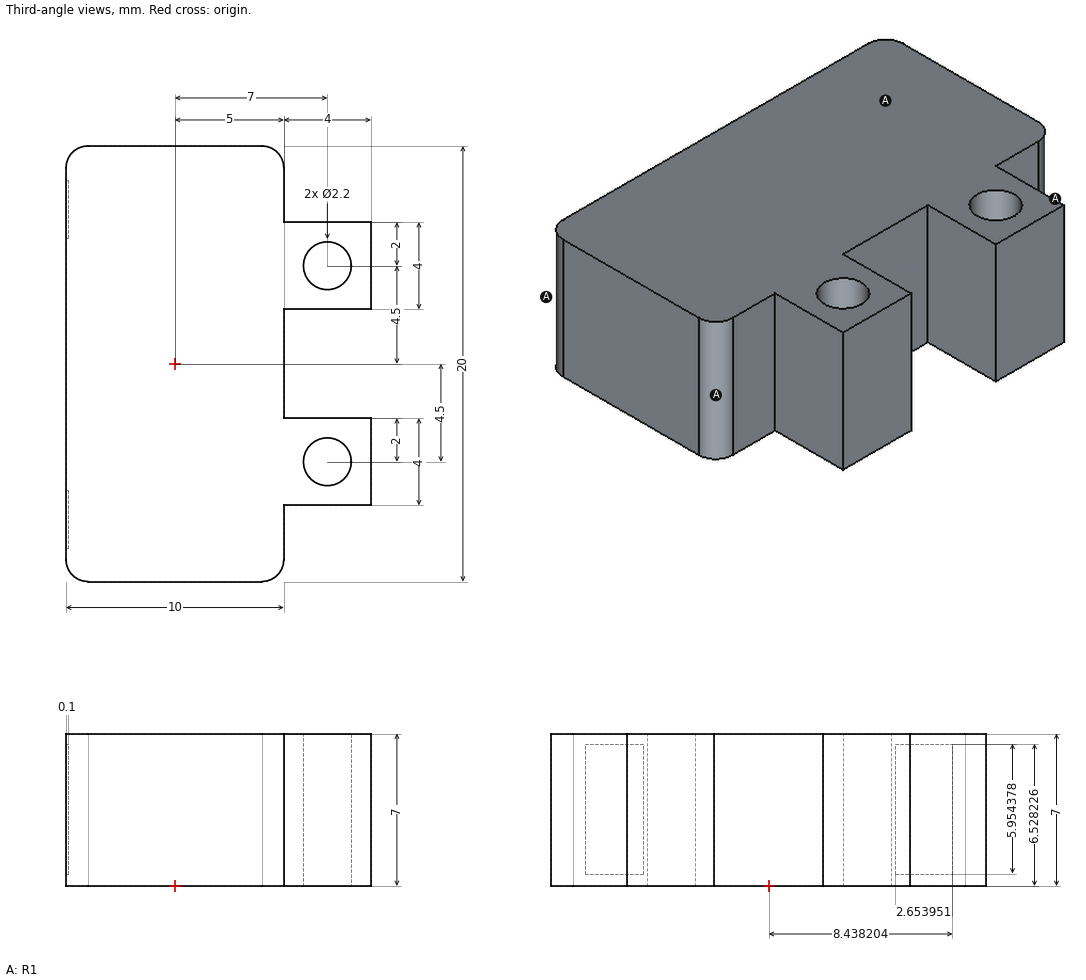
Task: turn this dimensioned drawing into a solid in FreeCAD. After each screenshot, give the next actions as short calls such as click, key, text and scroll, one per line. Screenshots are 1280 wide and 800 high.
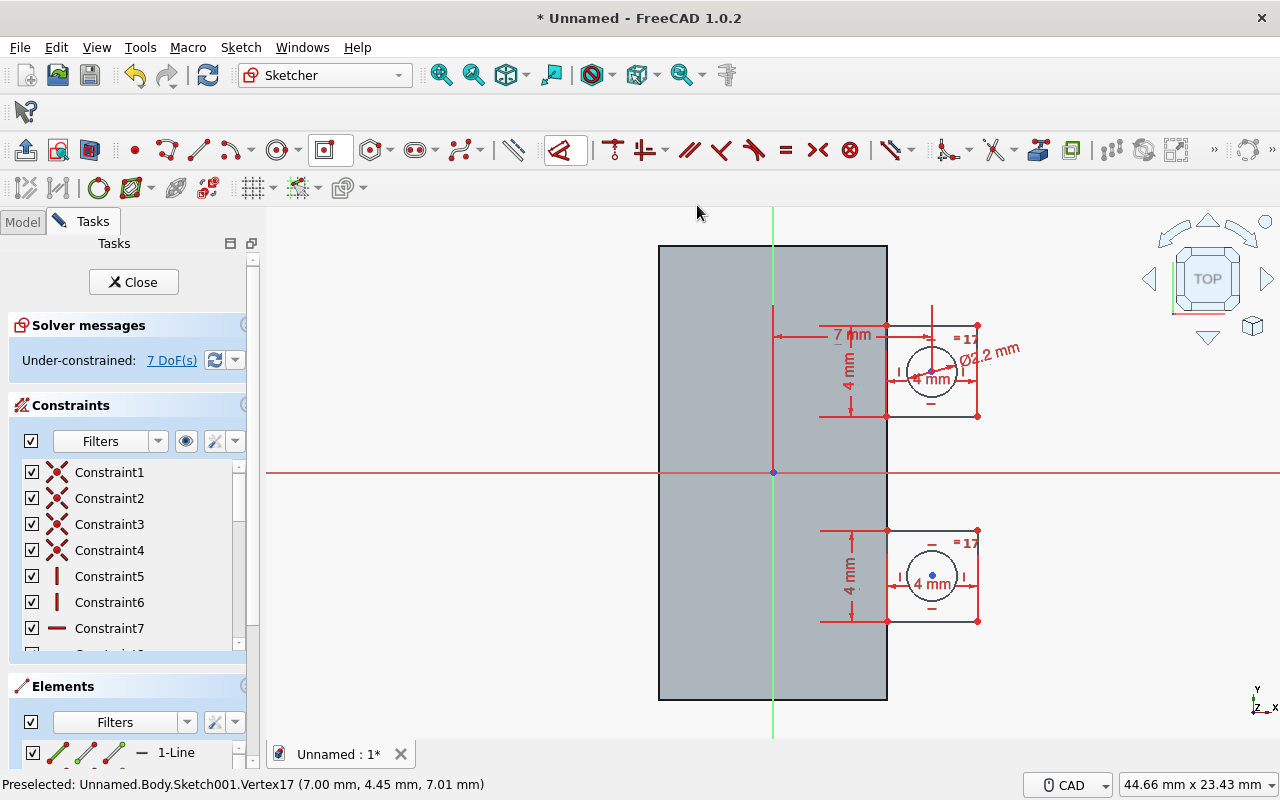
click(932, 576)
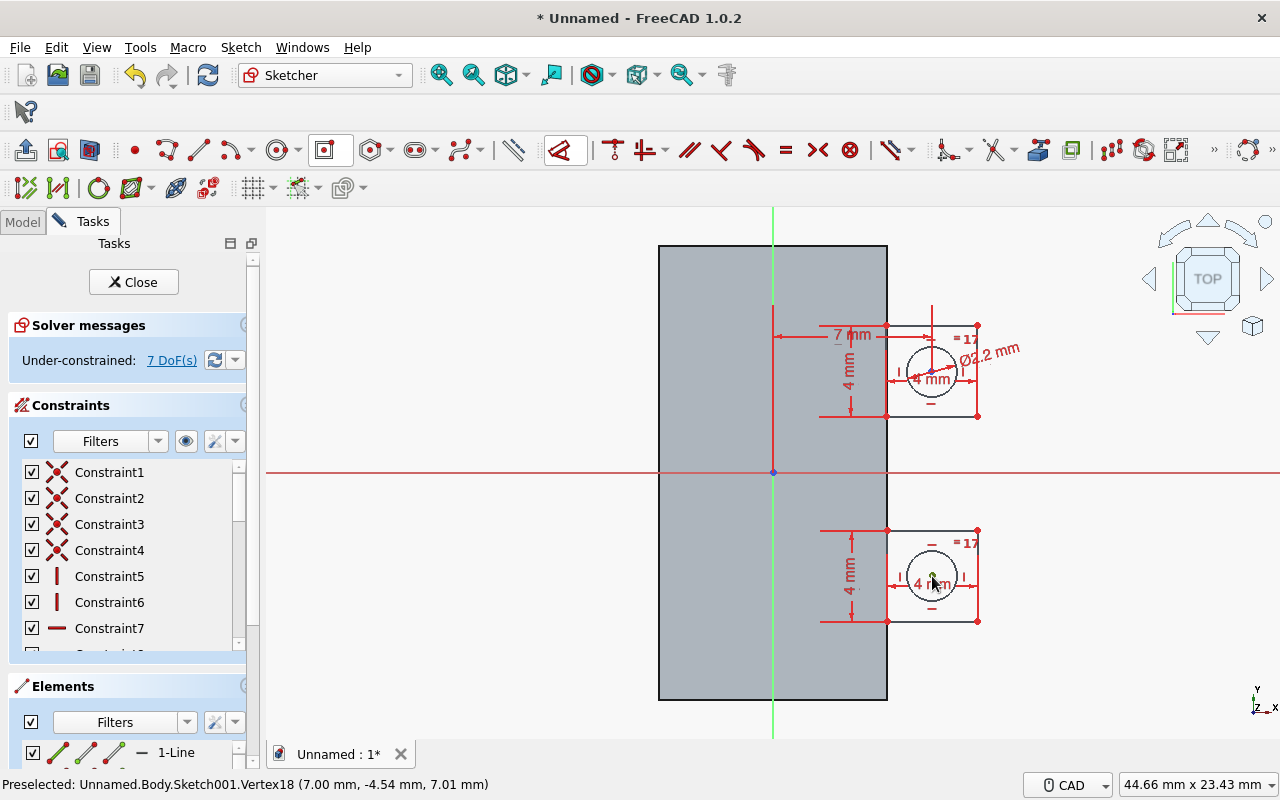
key(l)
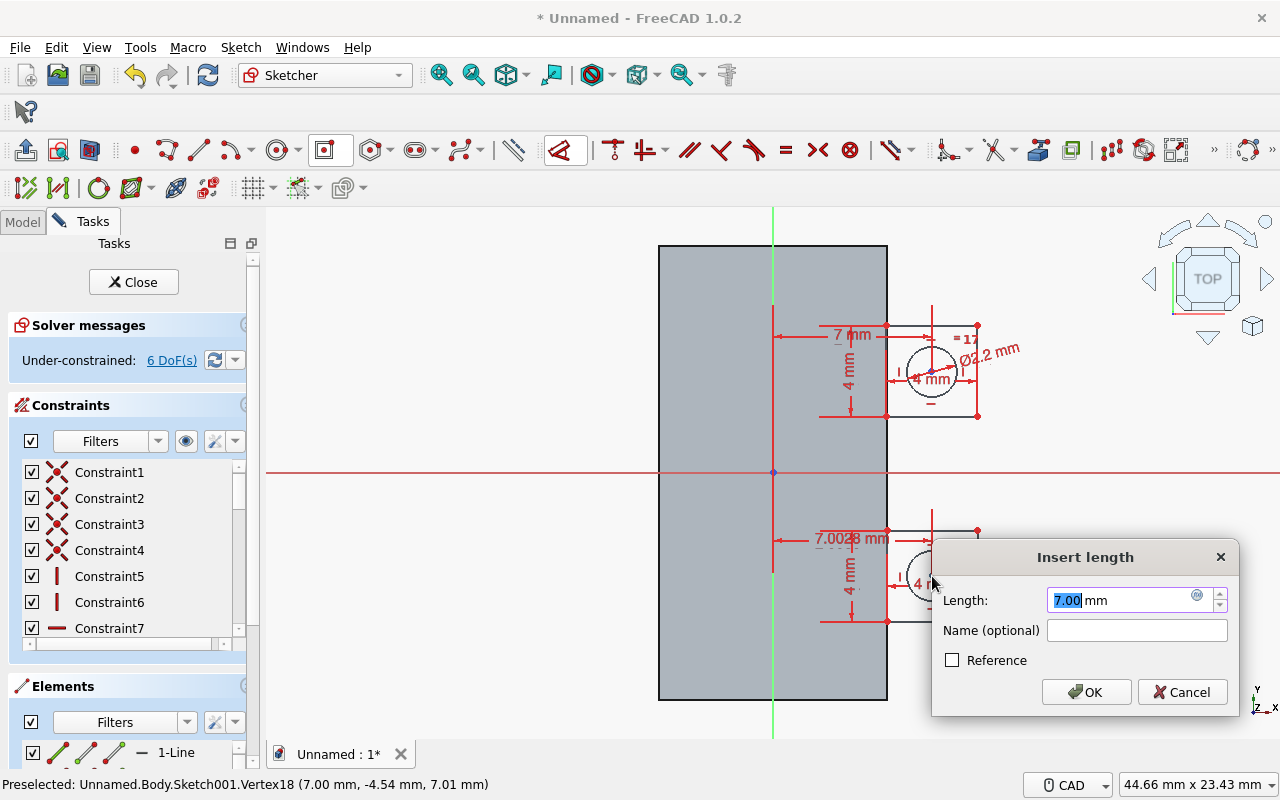
text(7)
key(Return)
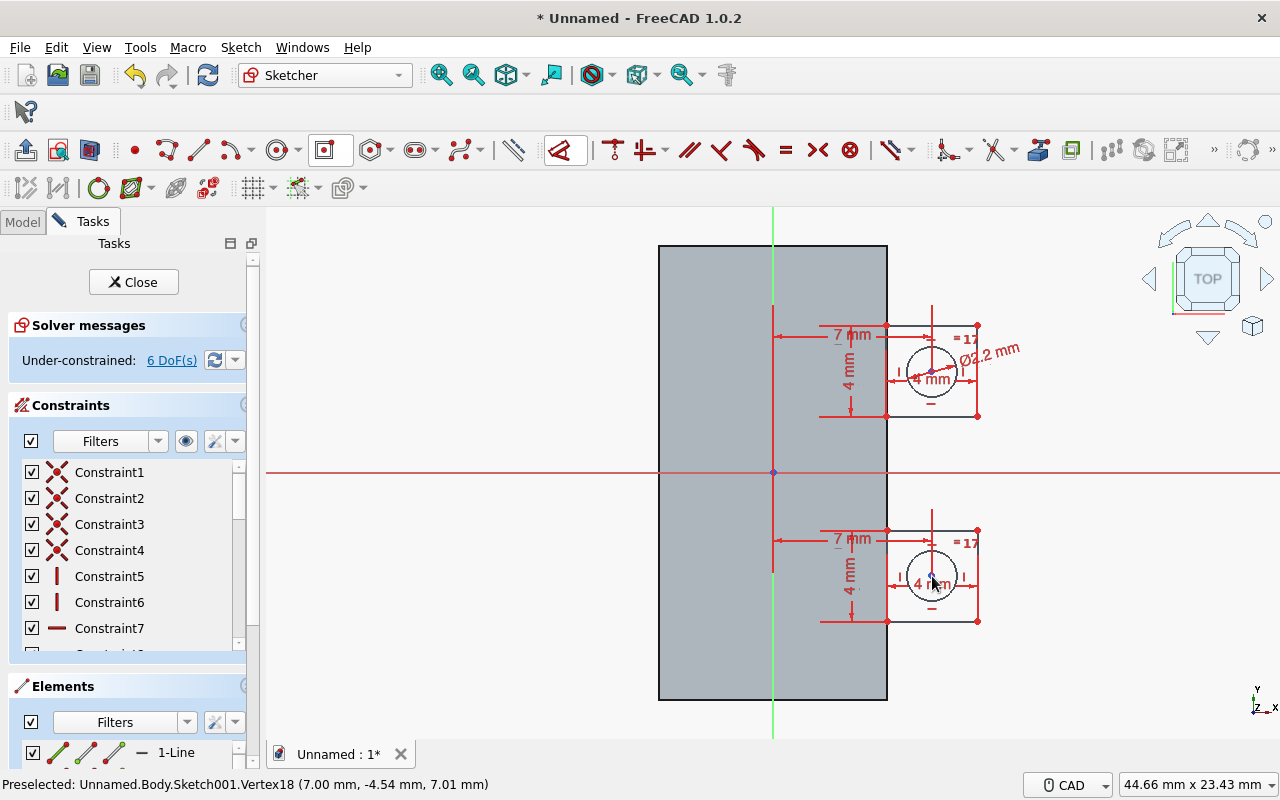
click(886, 326)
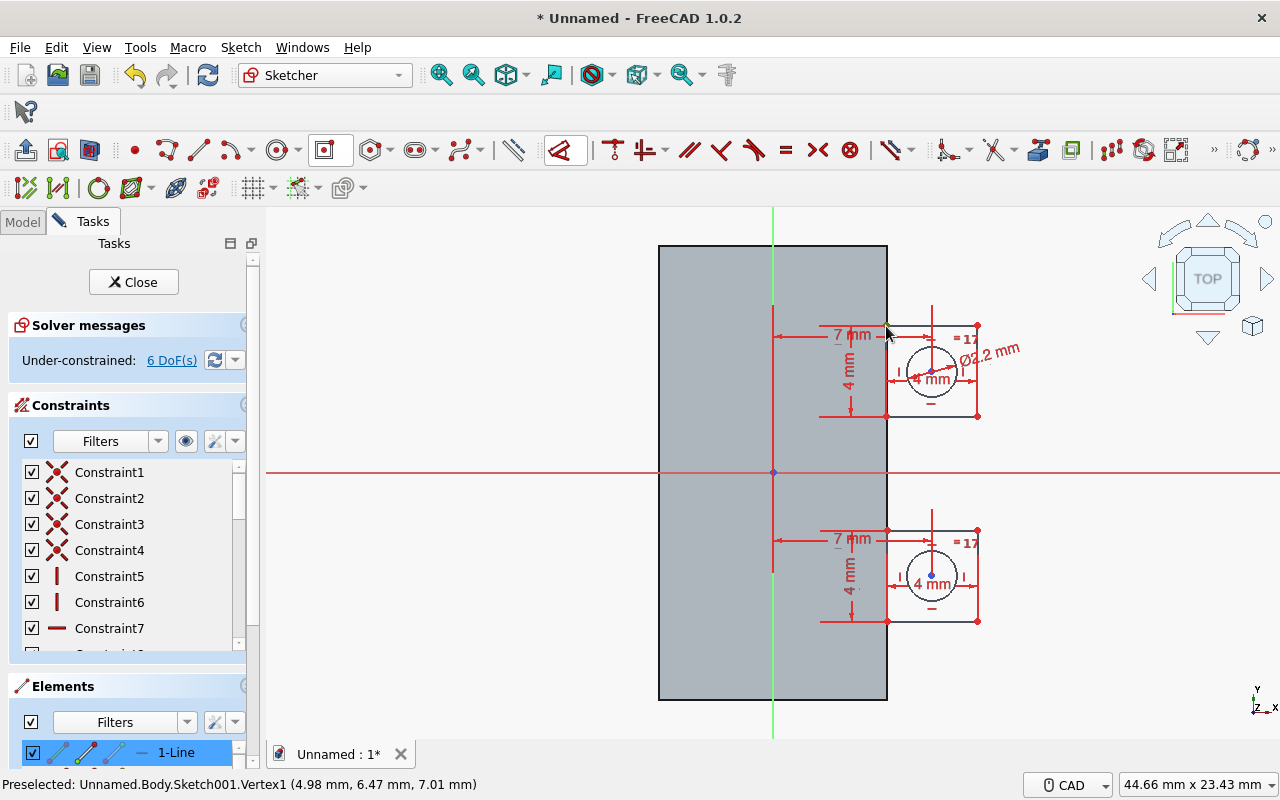
key(l)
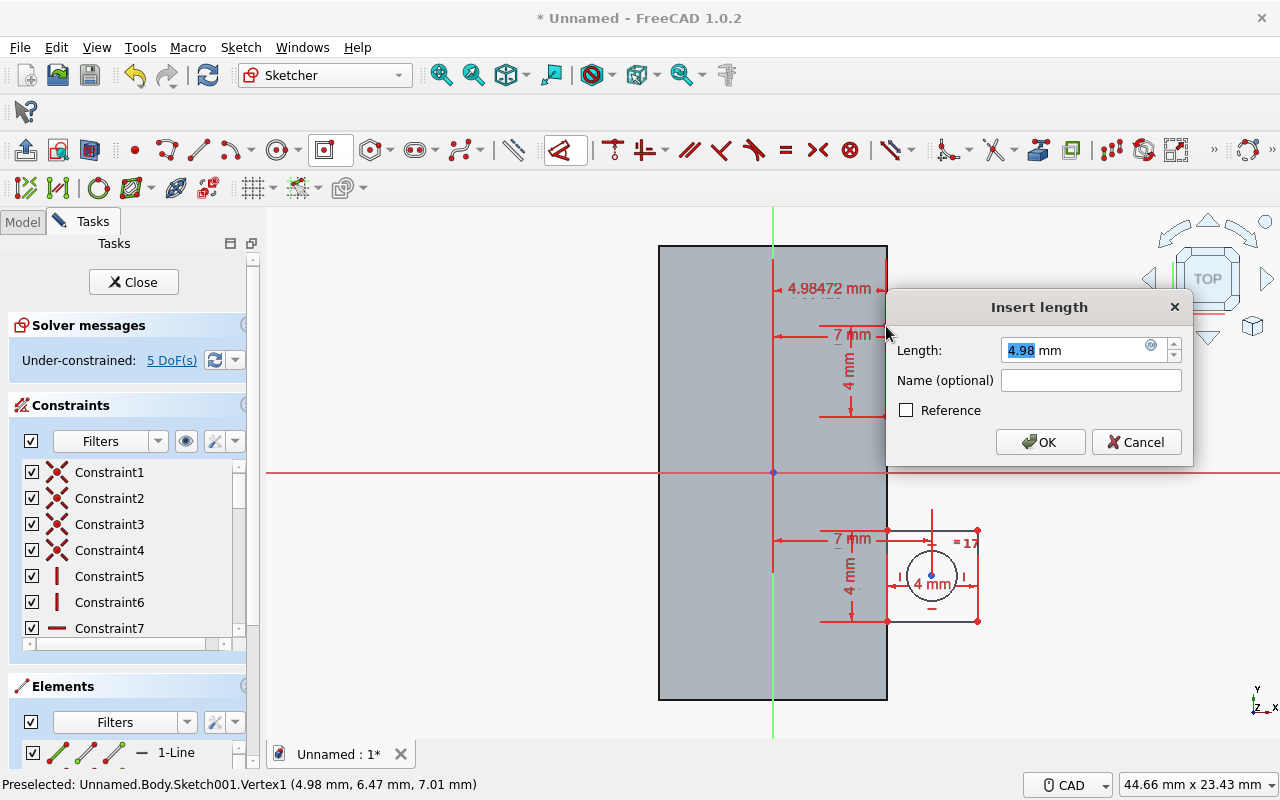
text(5)
key(Return)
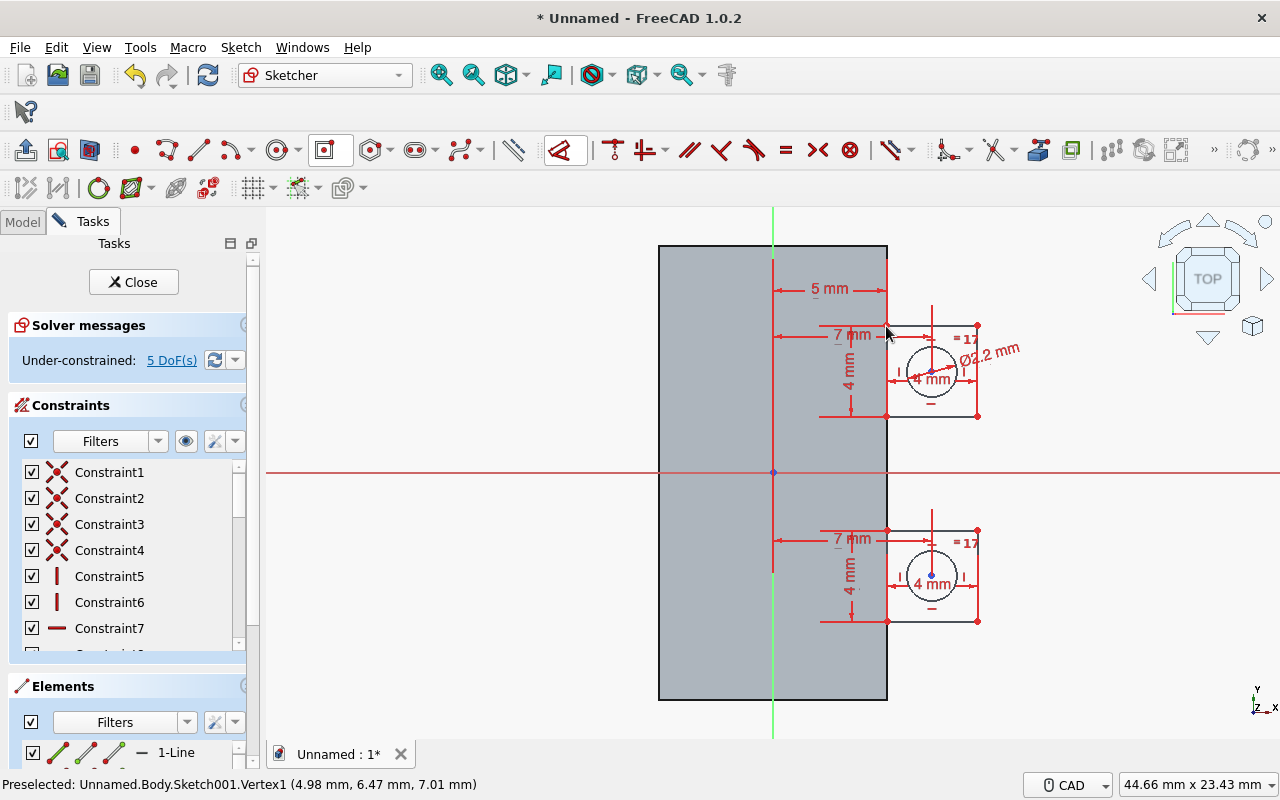
click(887, 531)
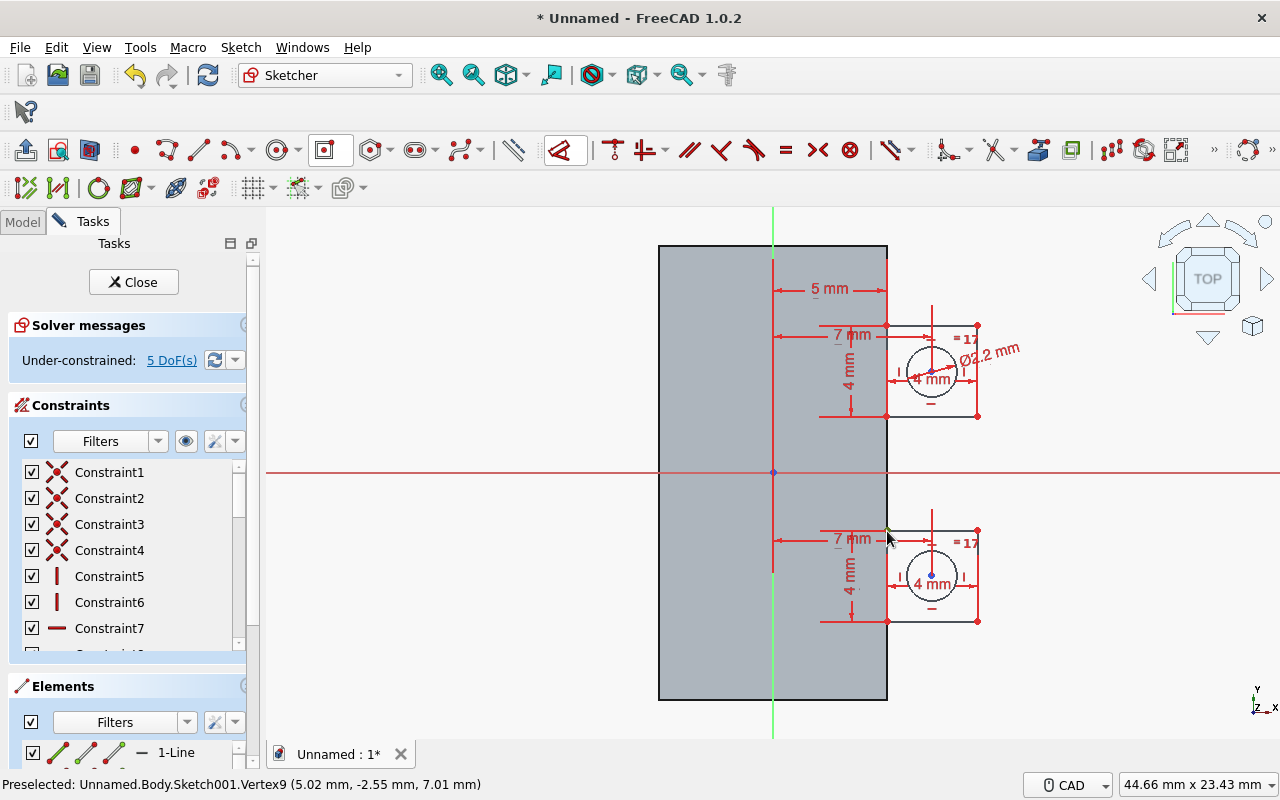
key(l)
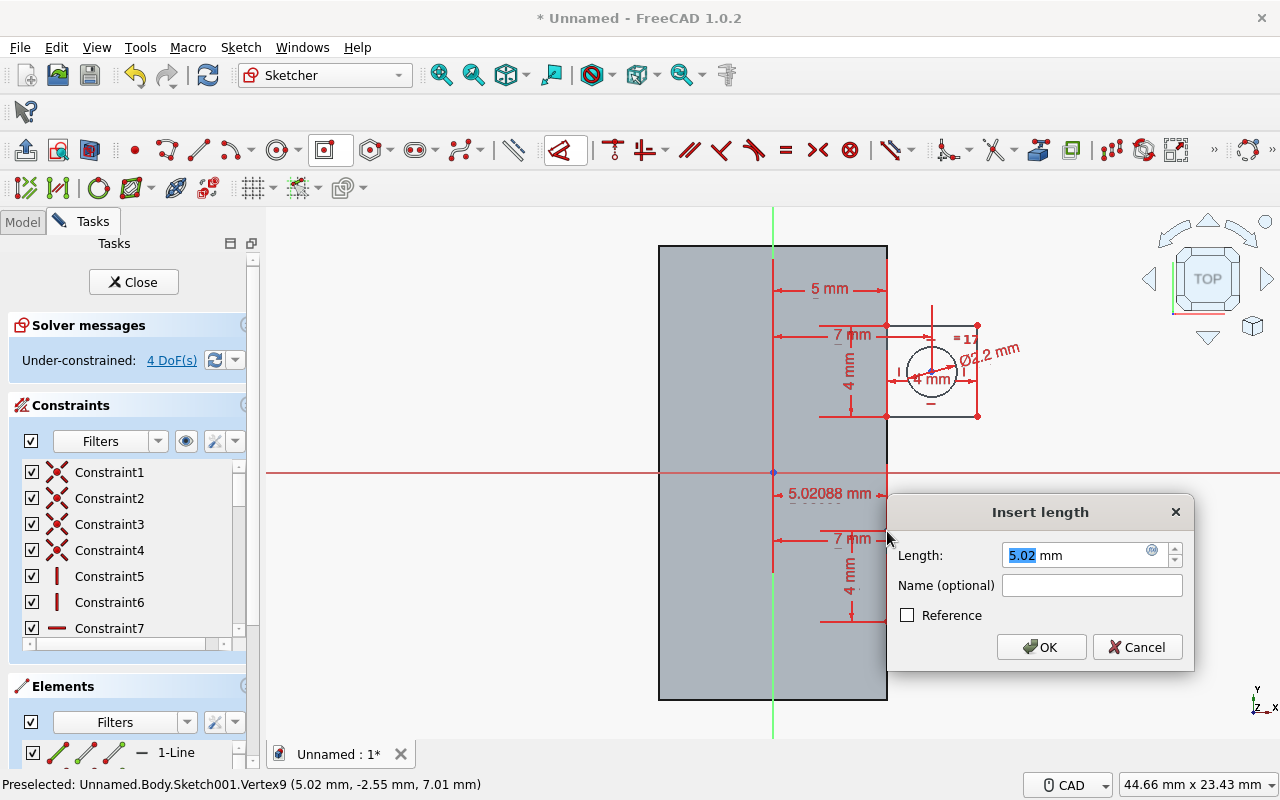
text(5)
key(Return)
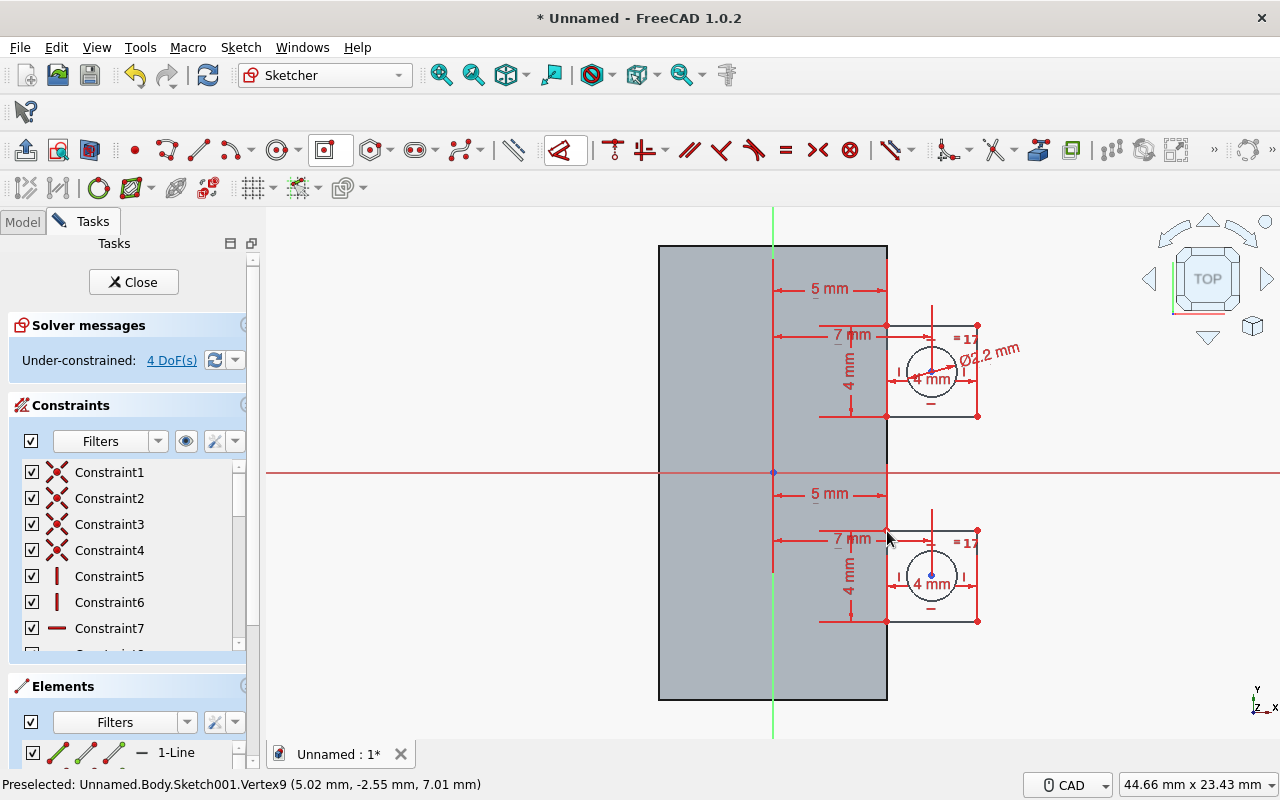
click(887, 326)